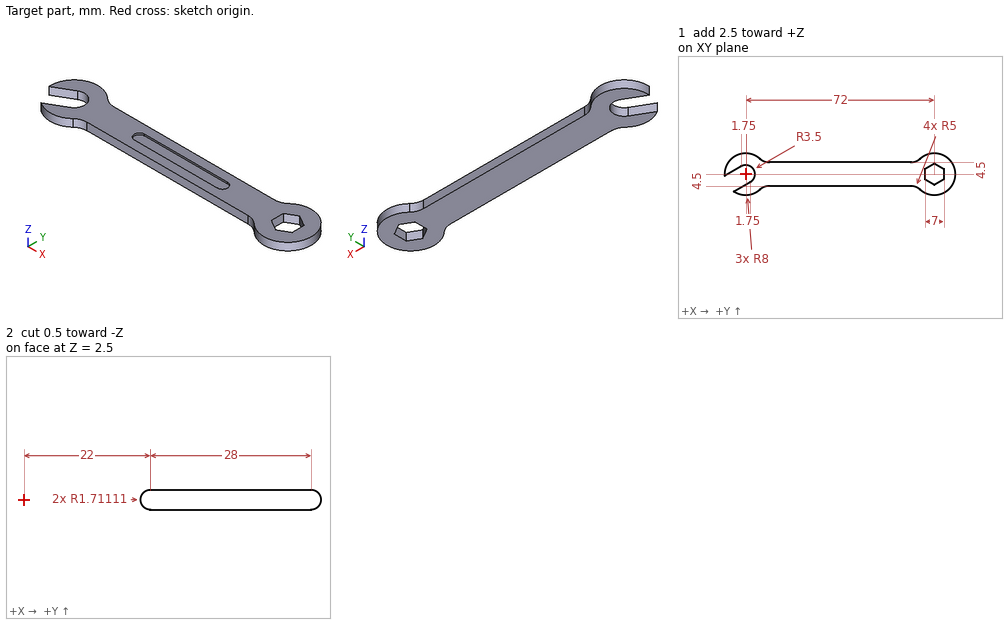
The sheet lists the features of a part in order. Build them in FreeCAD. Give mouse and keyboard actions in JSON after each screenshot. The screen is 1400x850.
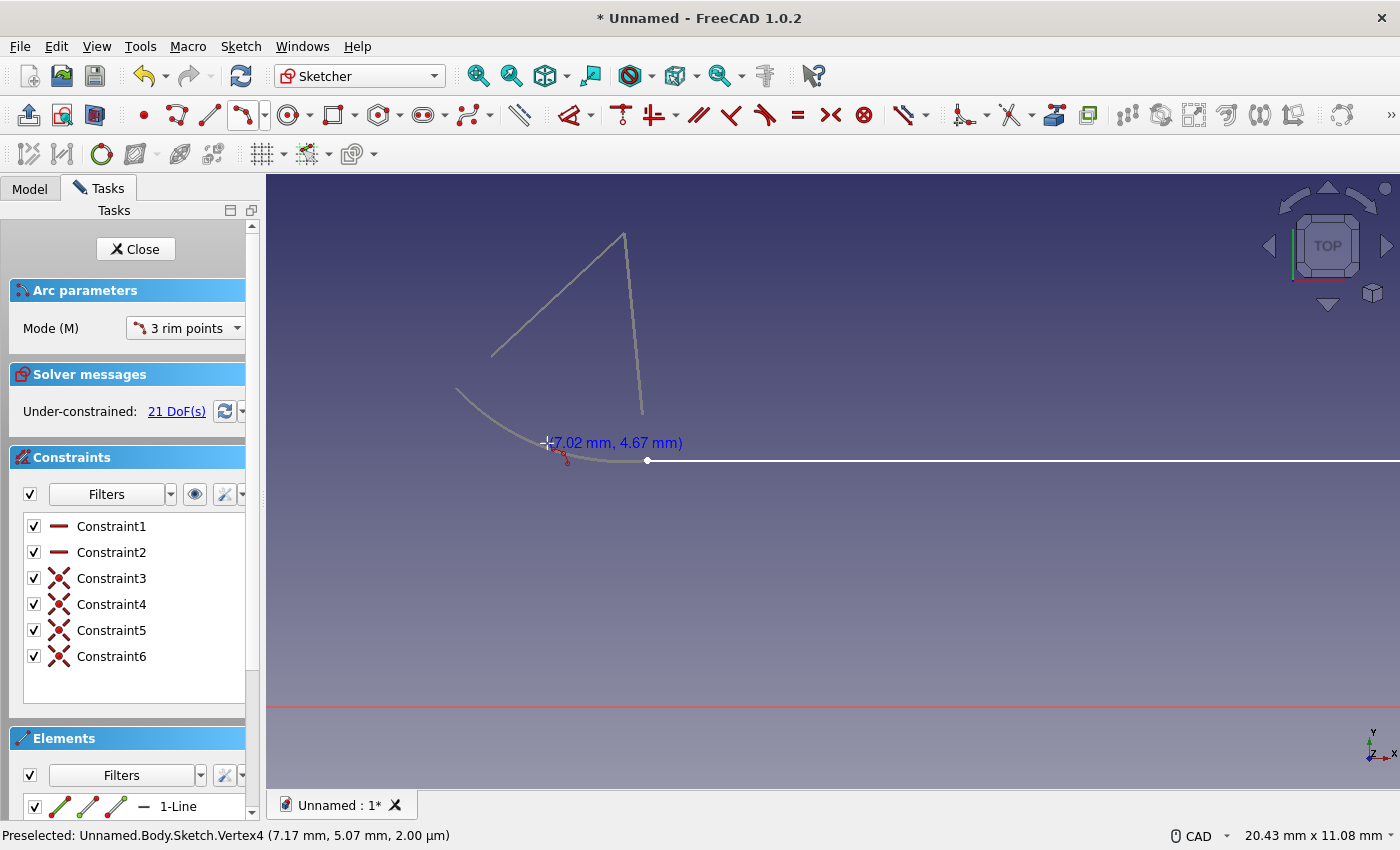
{"action": "left_click", "coordinate": [547, 437]}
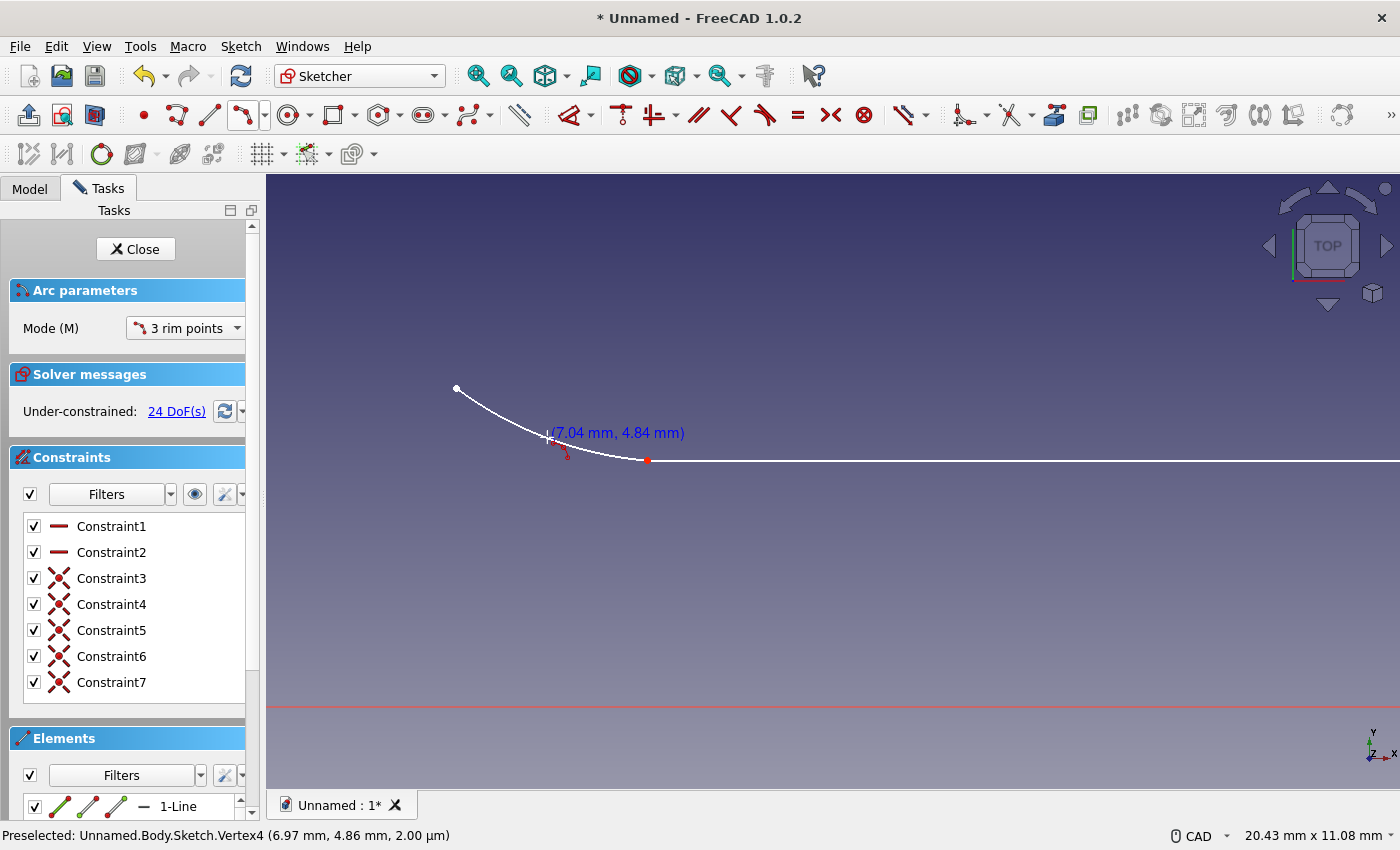
{"action": "scroll", "coordinate": [547, 443], "scroll_direction": "down", "scroll_amount": 10}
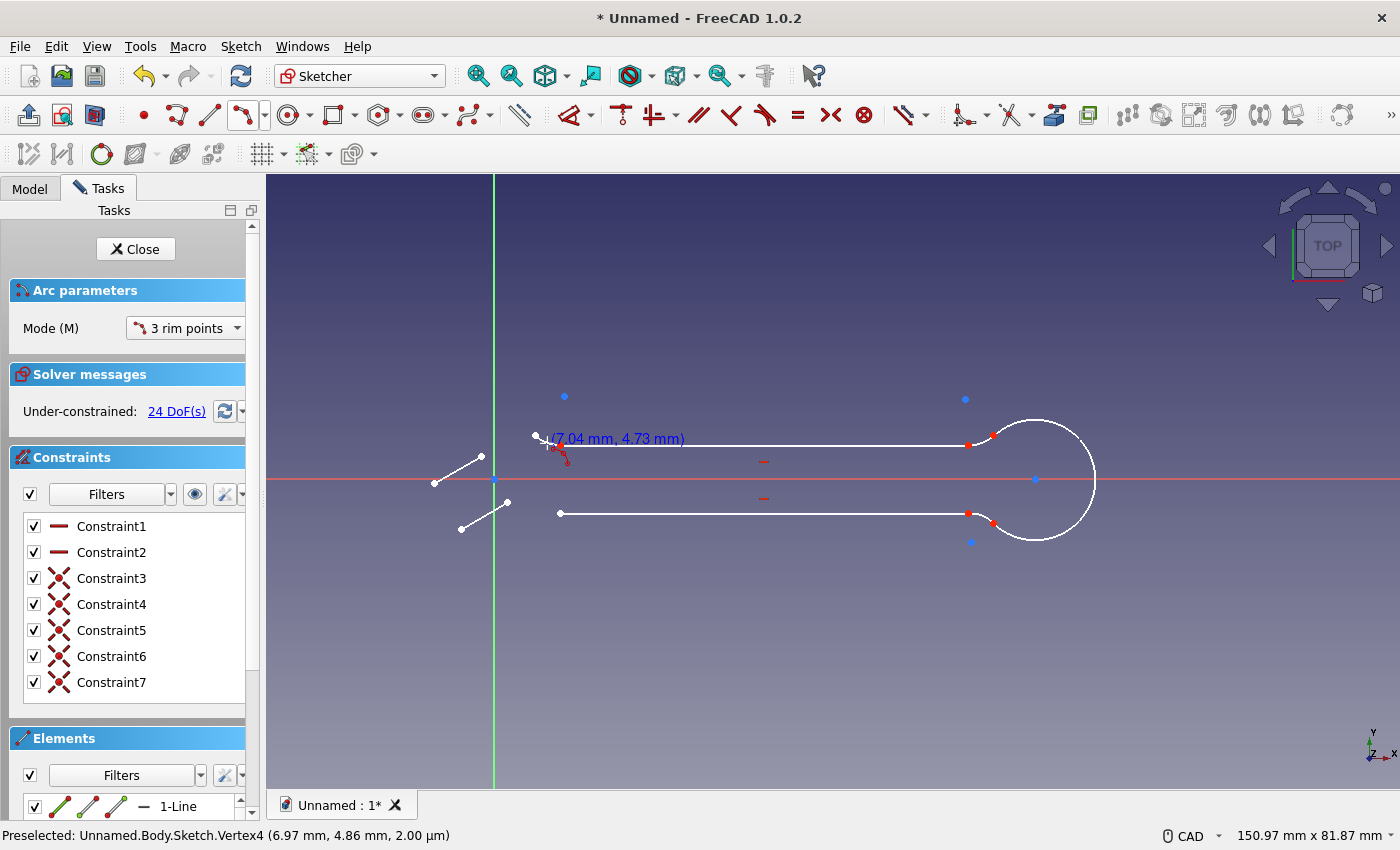
{"action": "left_click", "coordinate": [535, 436]}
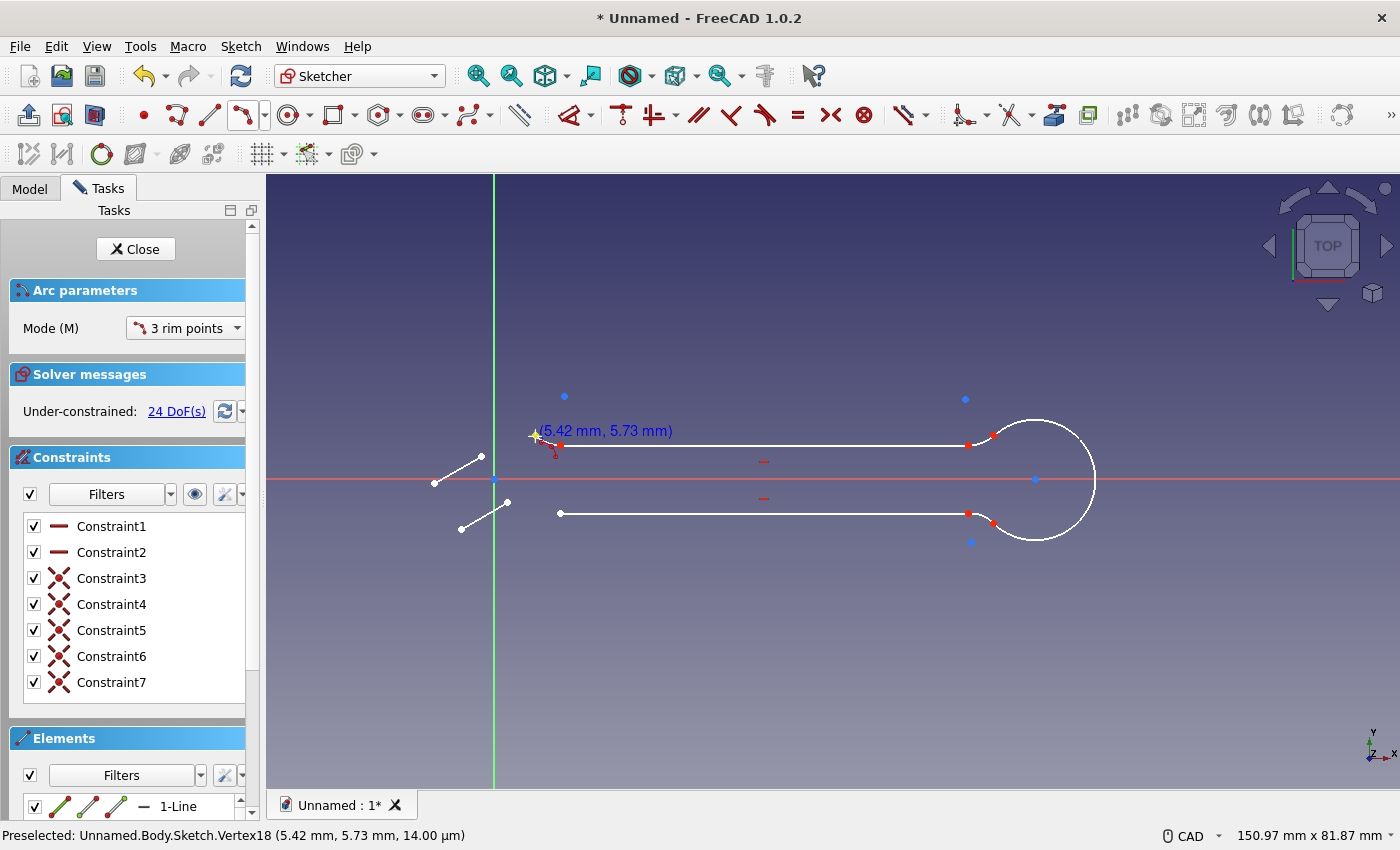
{"action": "scroll", "coordinate": [434, 483], "scroll_direction": "up", "scroll_amount": 7}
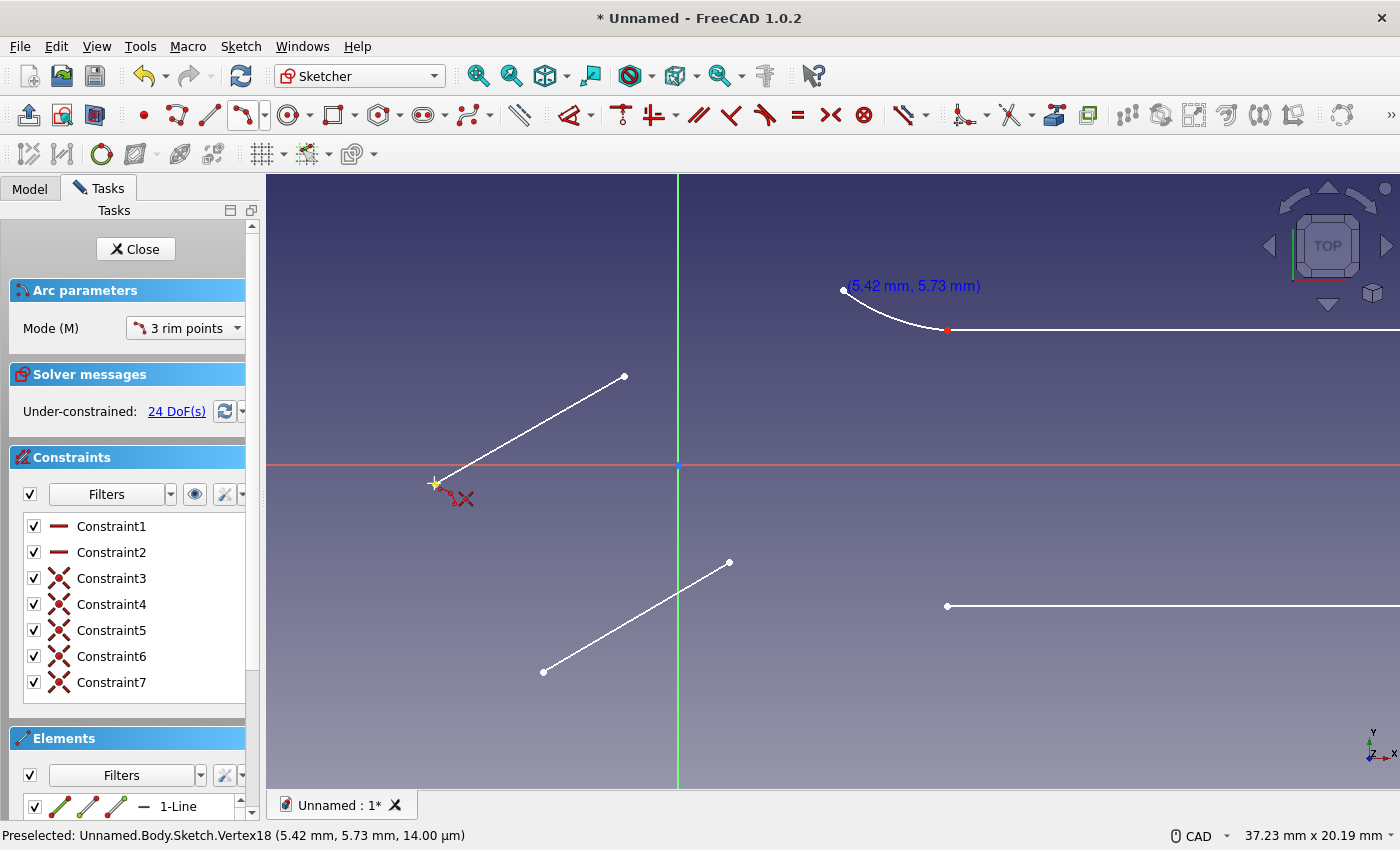
{"action": "left_click", "coordinate": [435, 484]}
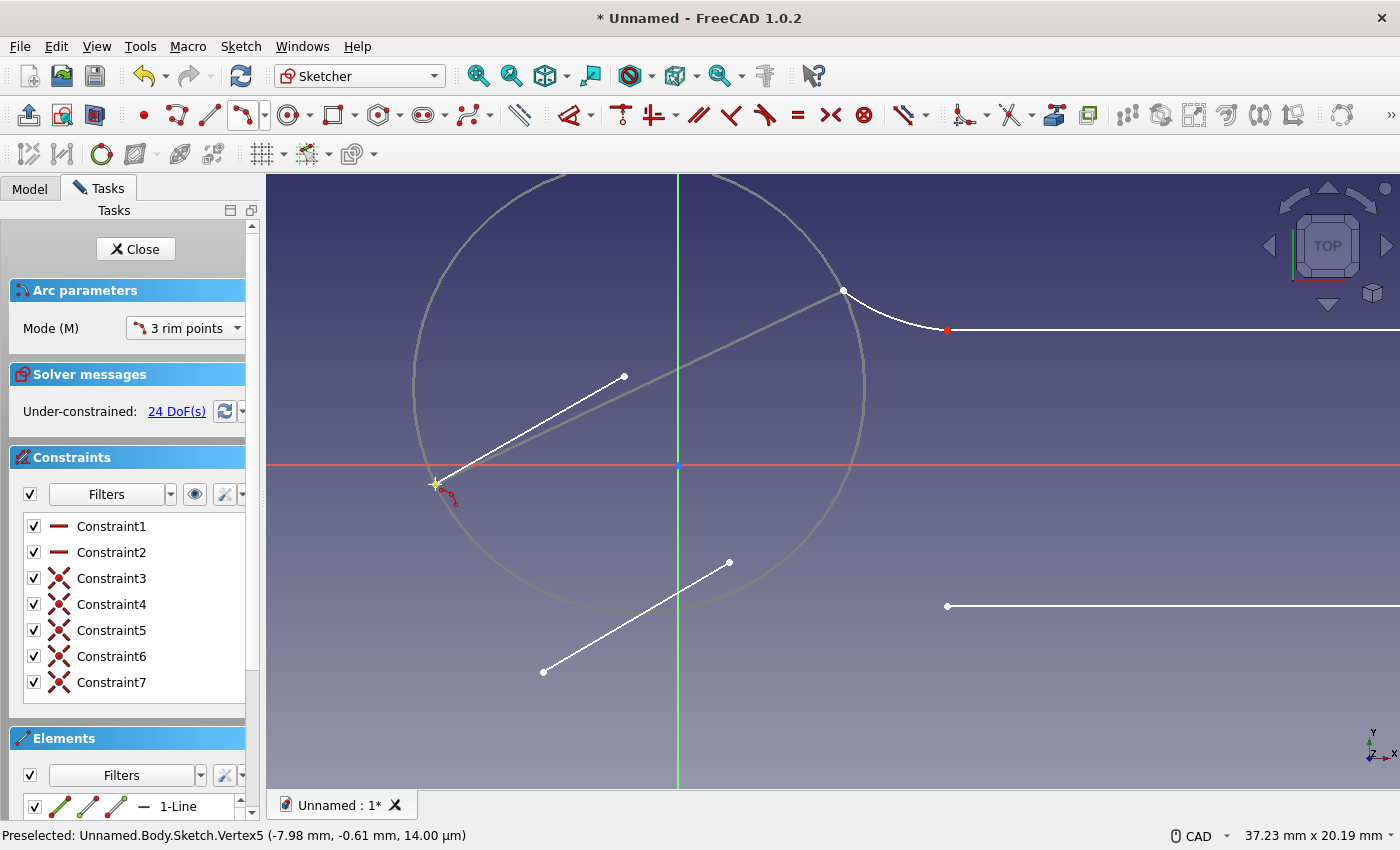
{"action": "scroll", "coordinate": [434, 483], "scroll_direction": "down", "scroll_amount": 7}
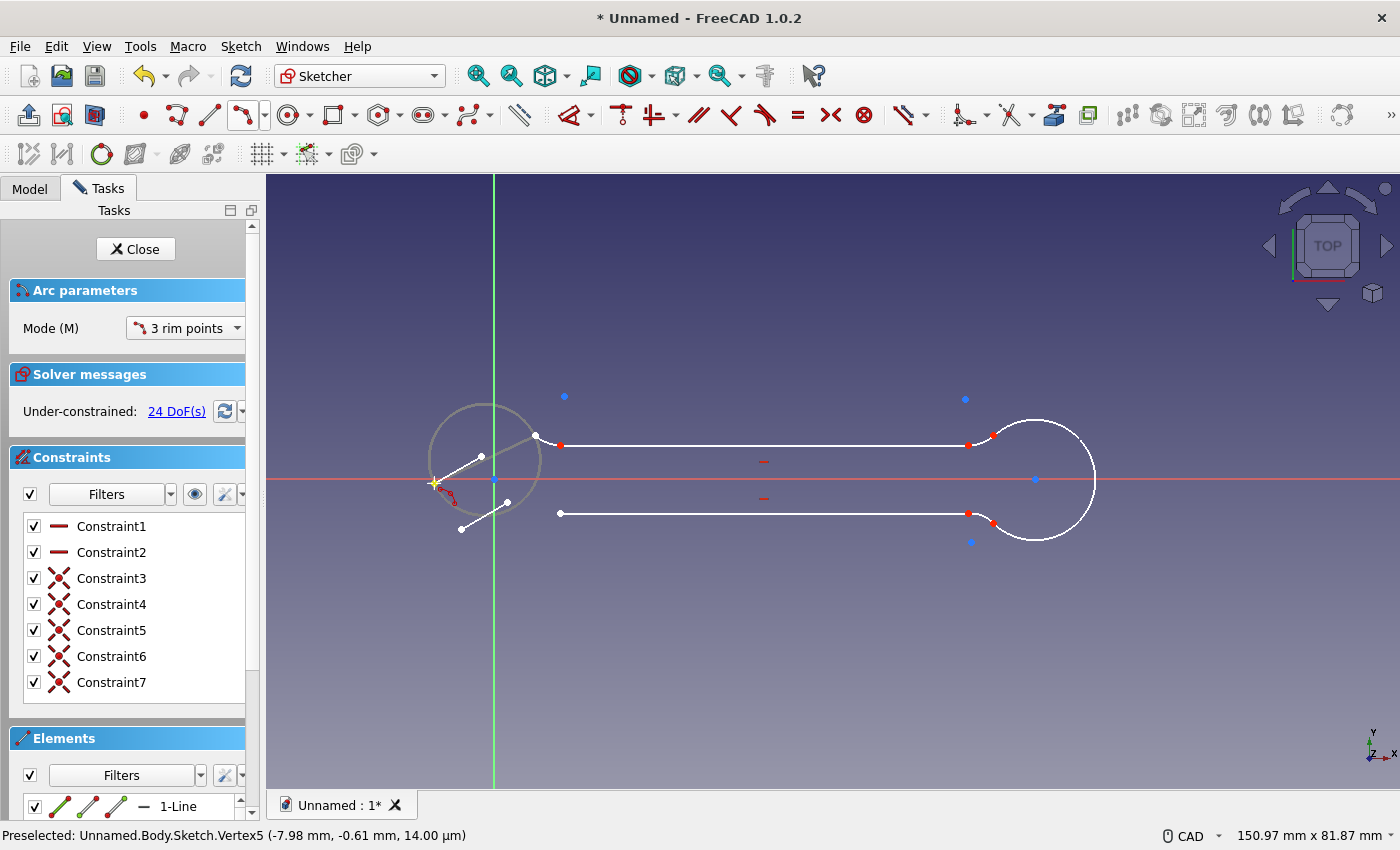
{"action": "left_click", "coordinate": [468, 425]}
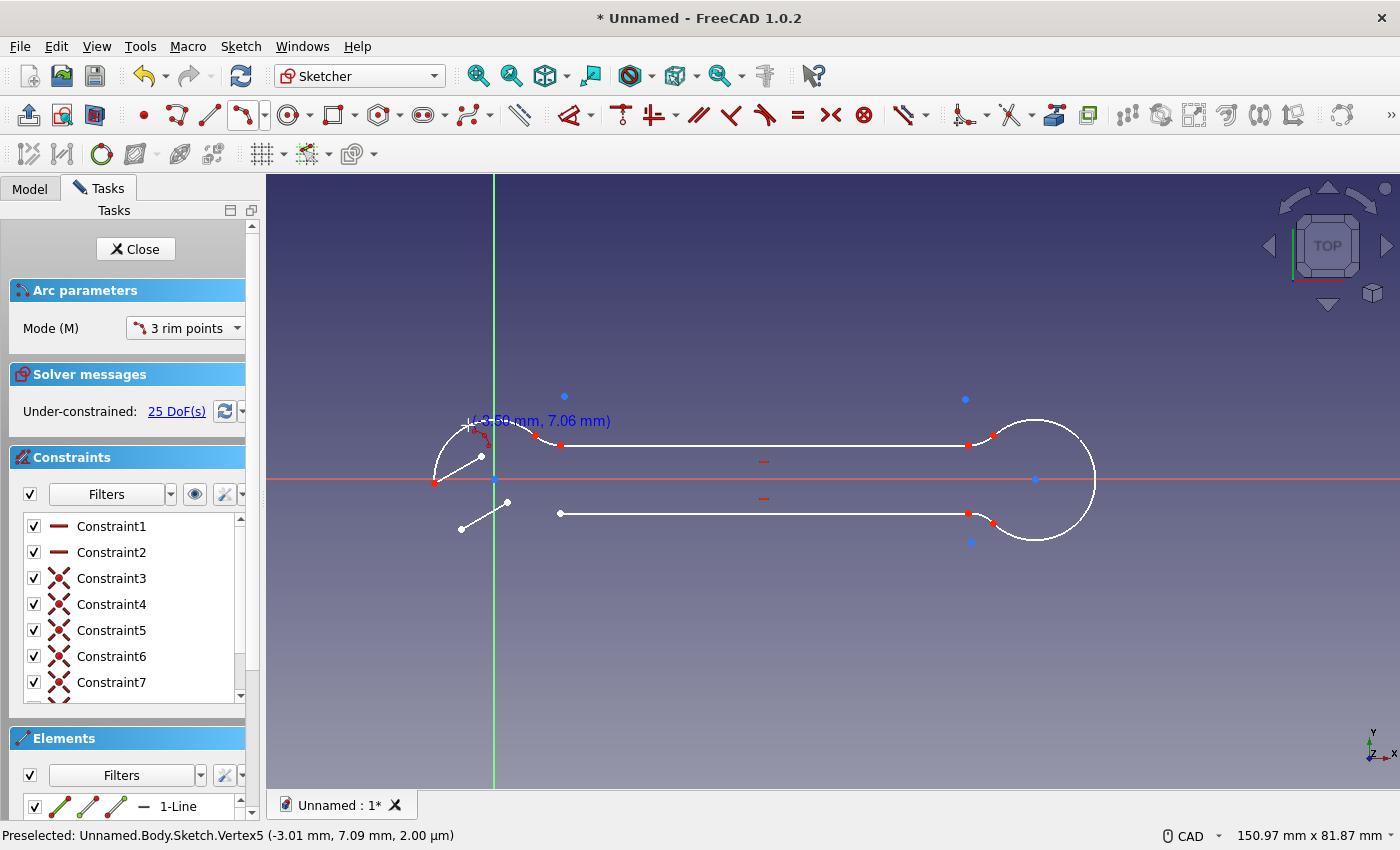
{"action": "left_click", "coordinate": [481, 457]}
{"action": "left_click", "coordinate": [507, 503]}
{"action": "left_click", "coordinate": [512, 460]}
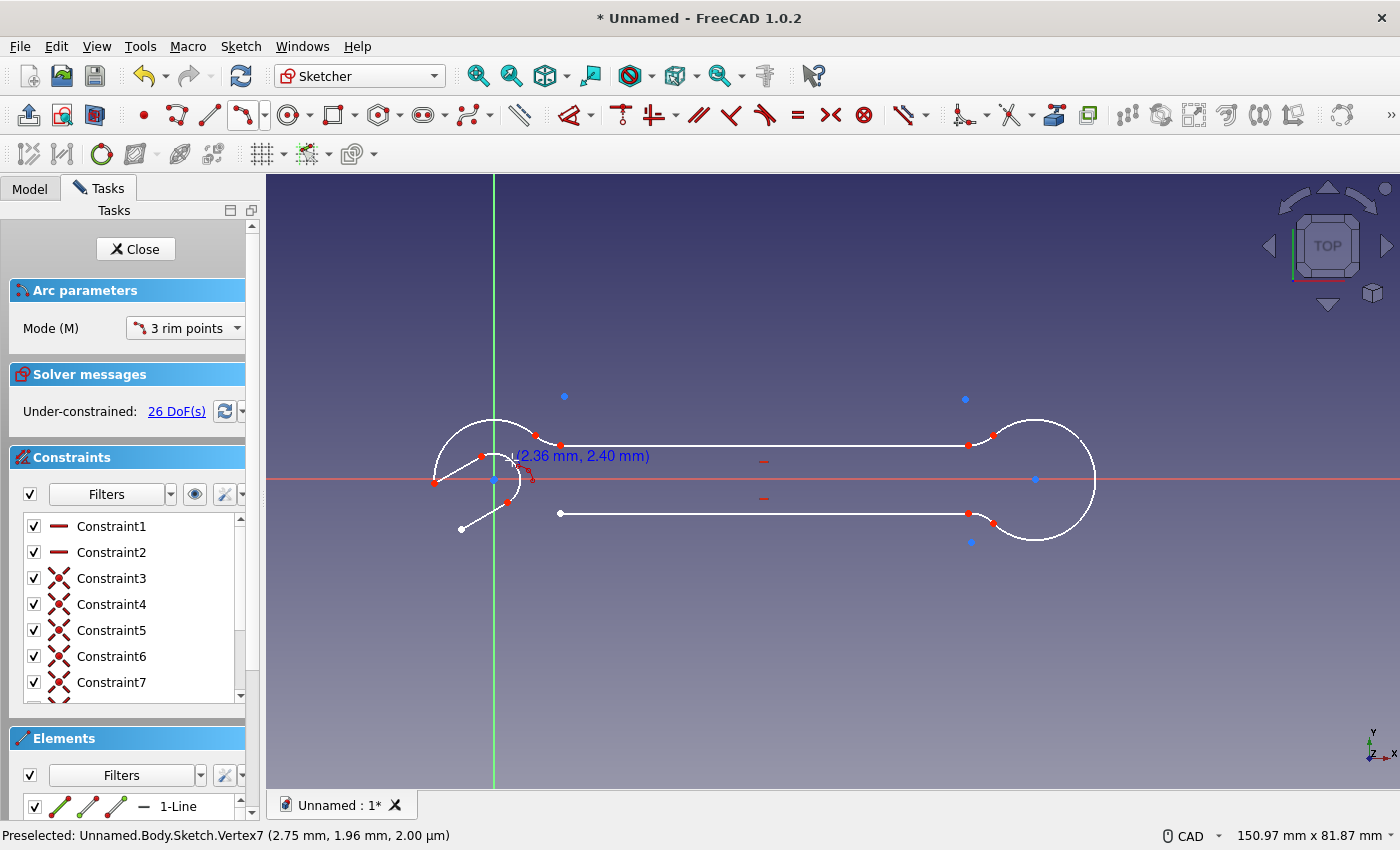
{"action": "left_click", "coordinate": [461, 530]}
{"action": "left_click", "coordinate": [535, 523]}